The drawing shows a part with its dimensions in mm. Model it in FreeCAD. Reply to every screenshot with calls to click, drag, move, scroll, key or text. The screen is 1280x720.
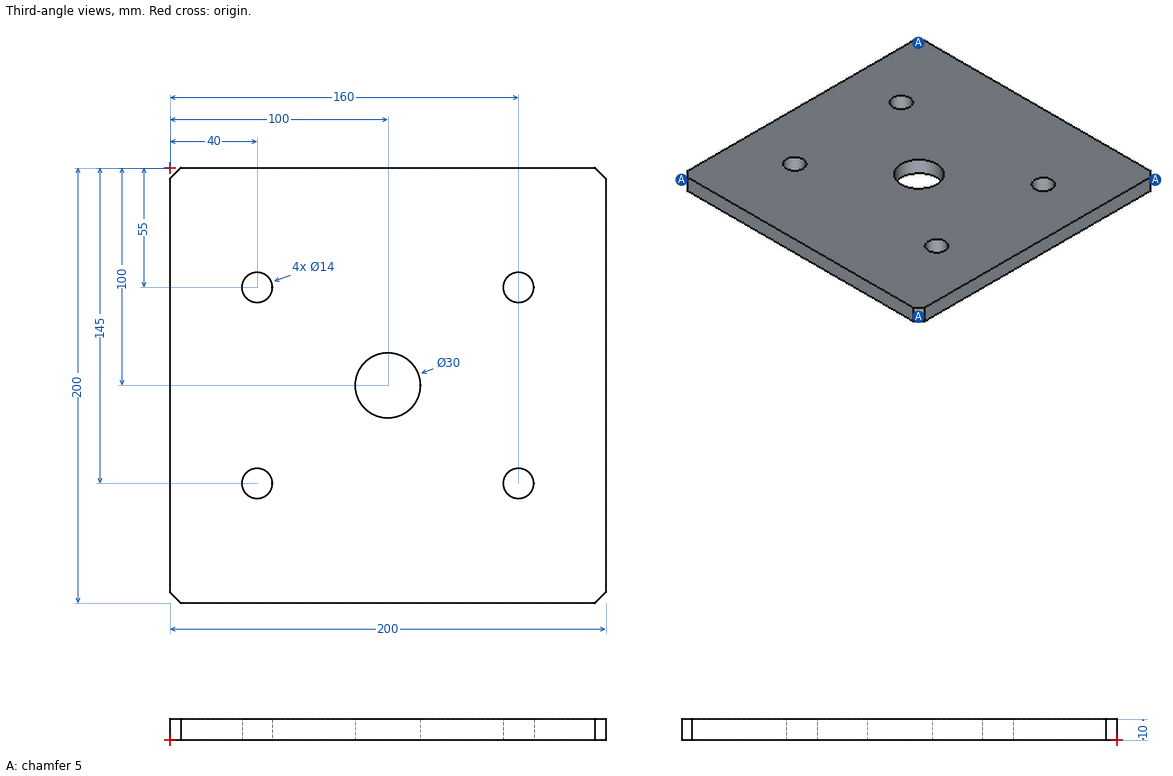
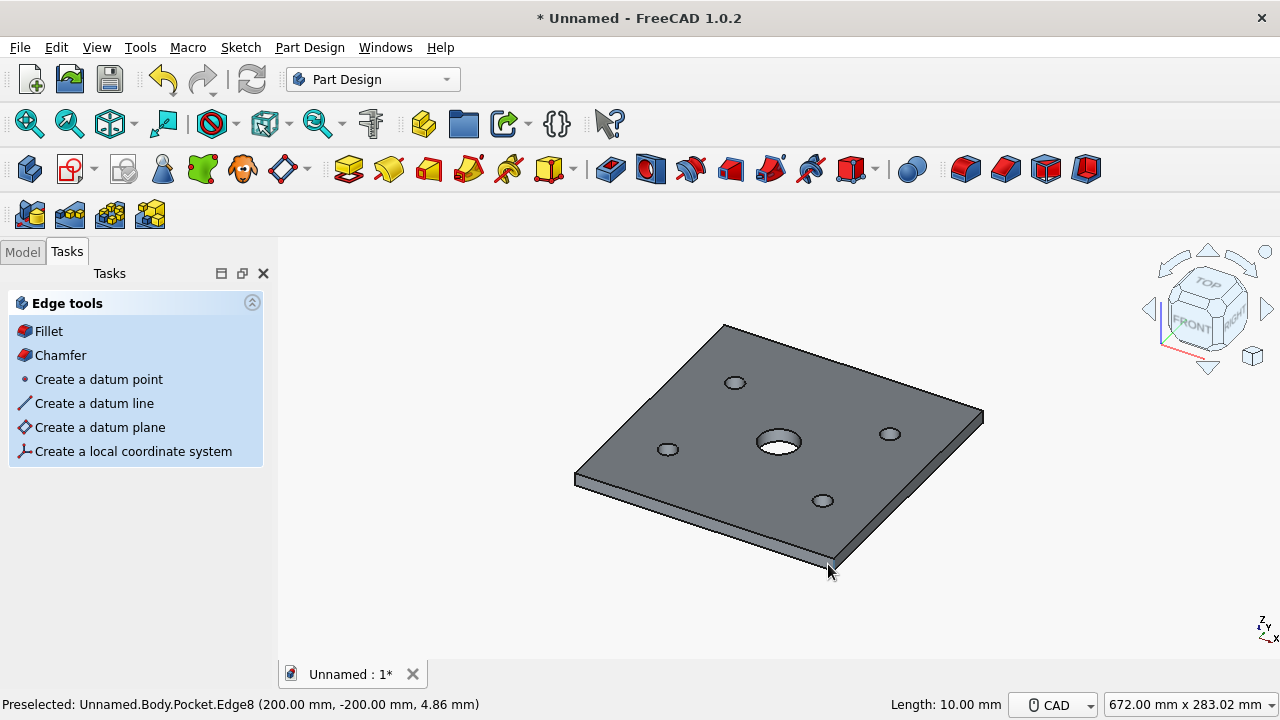
scroll(724, 330, up, 5)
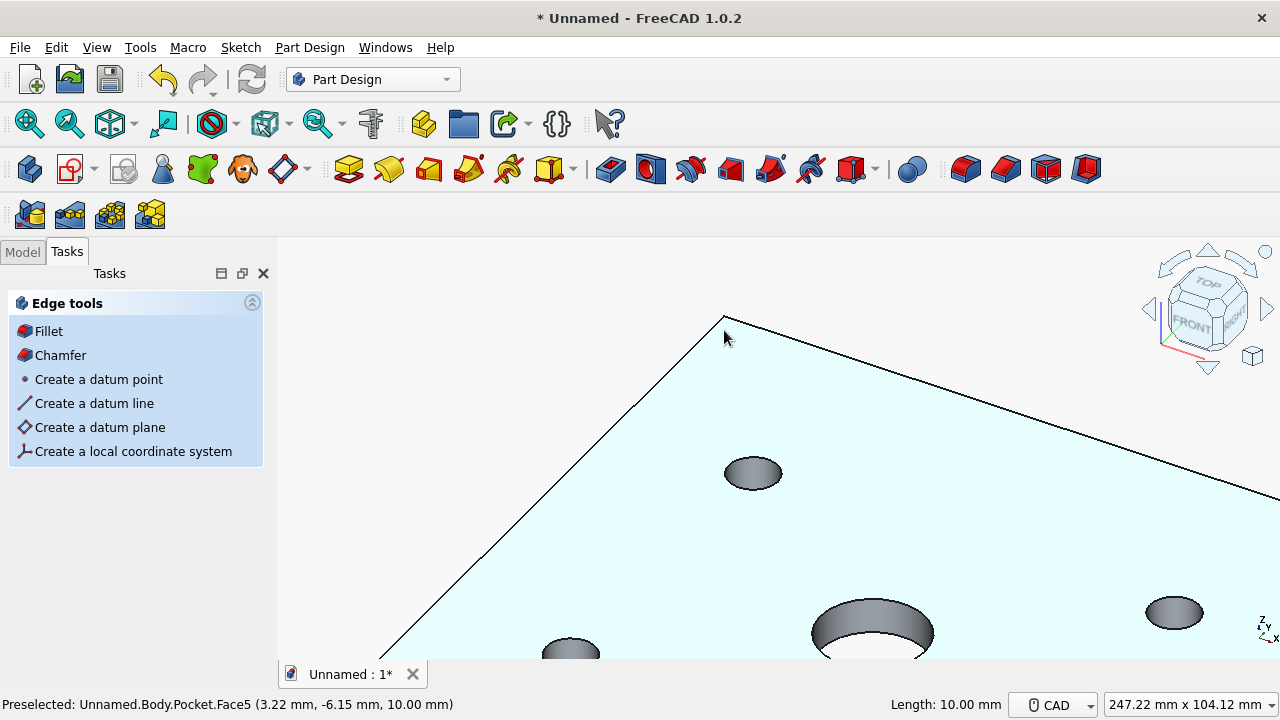
click(30, 124)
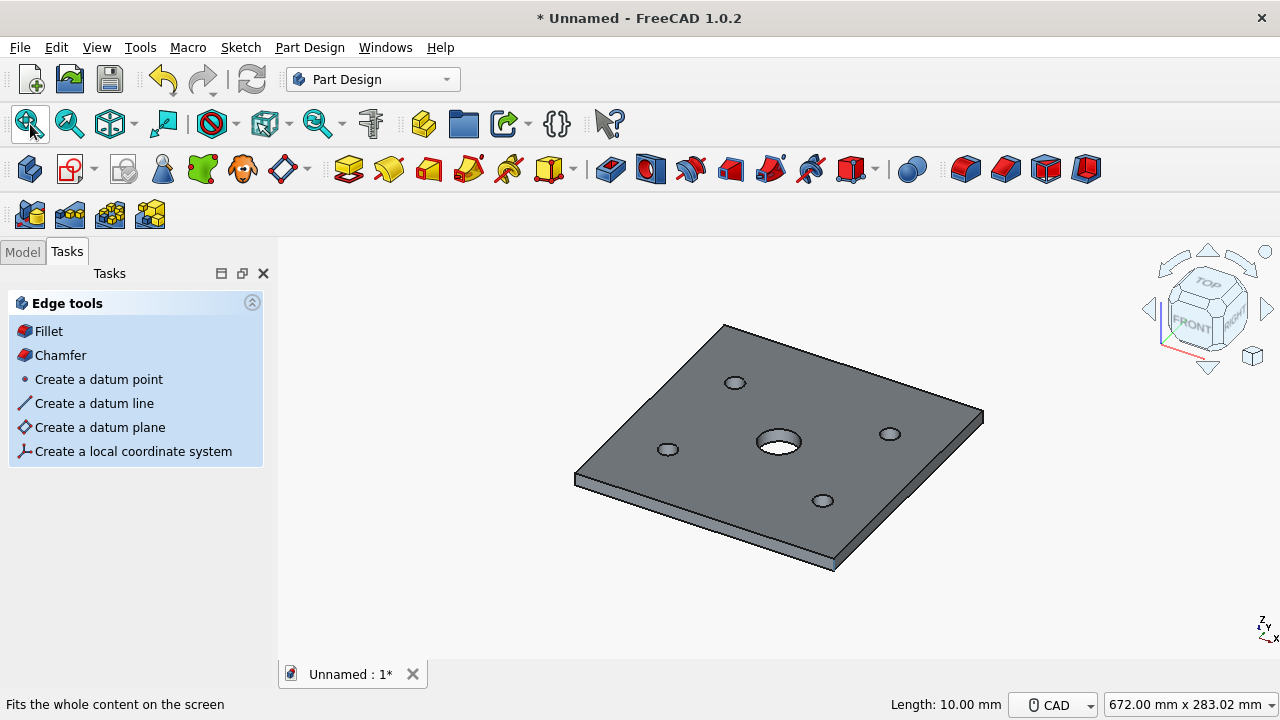
key(0)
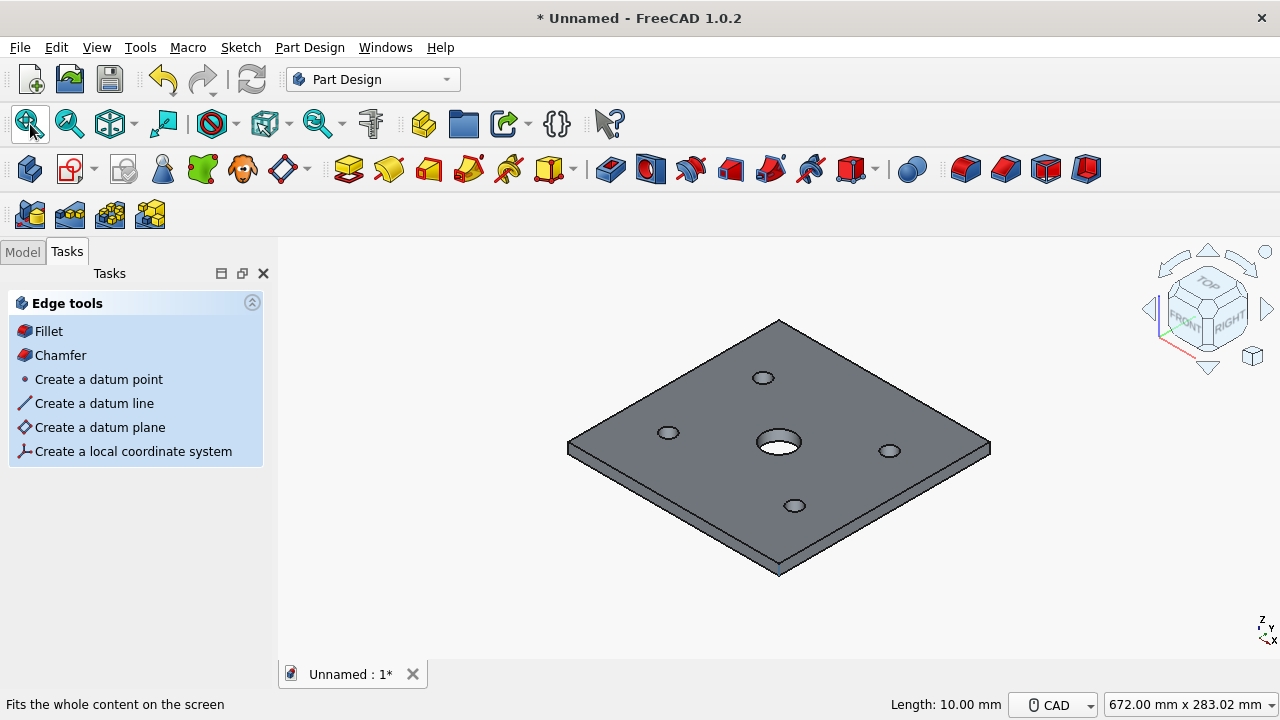
scroll(779, 325, up, 5)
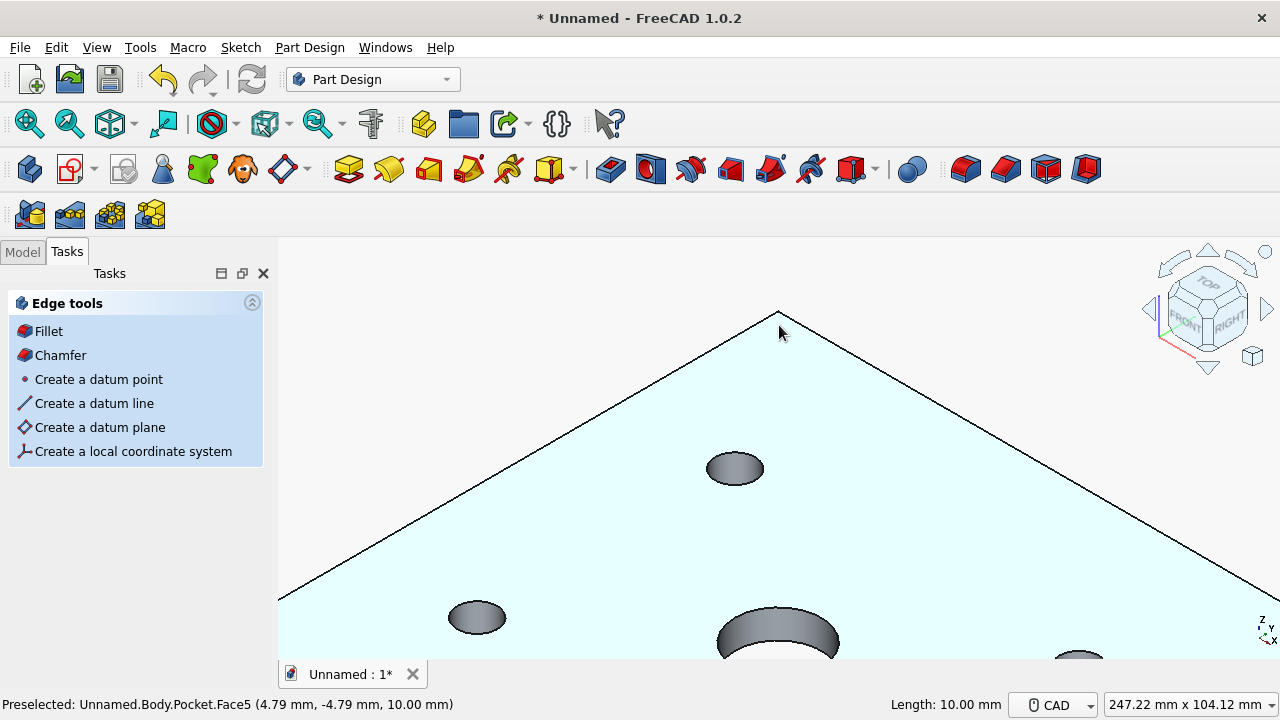
click(30, 124)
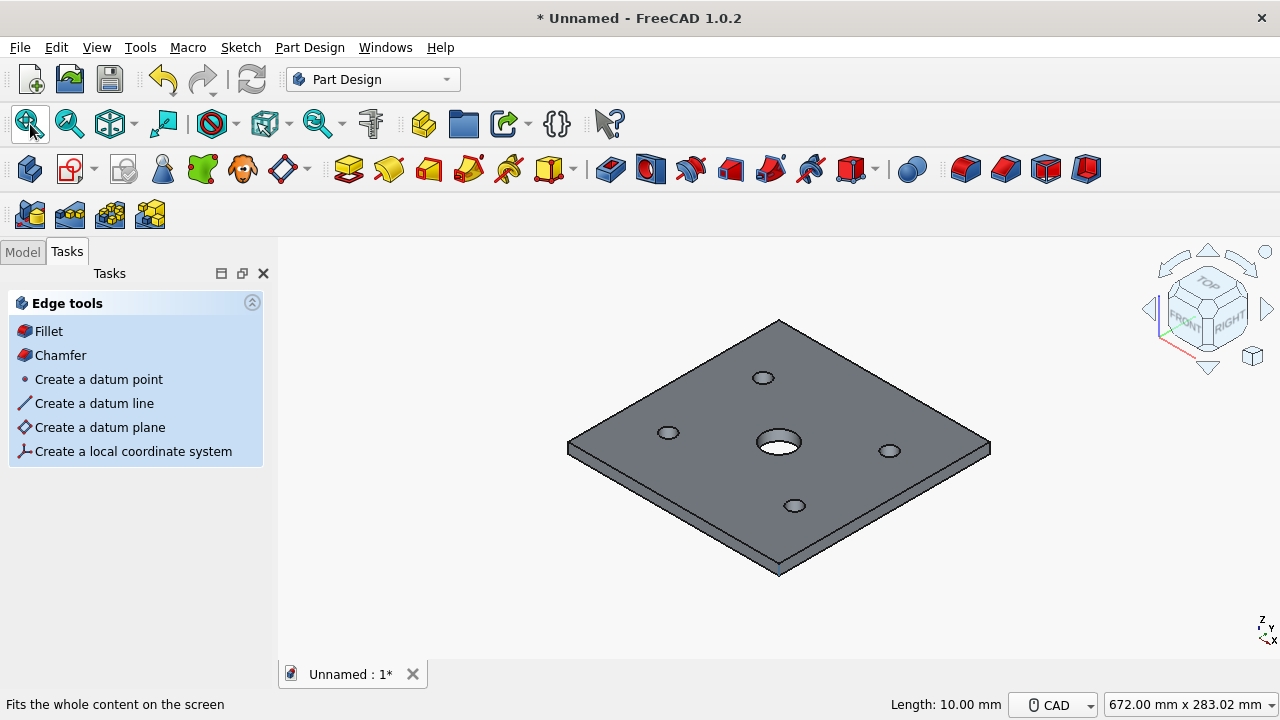
key(2)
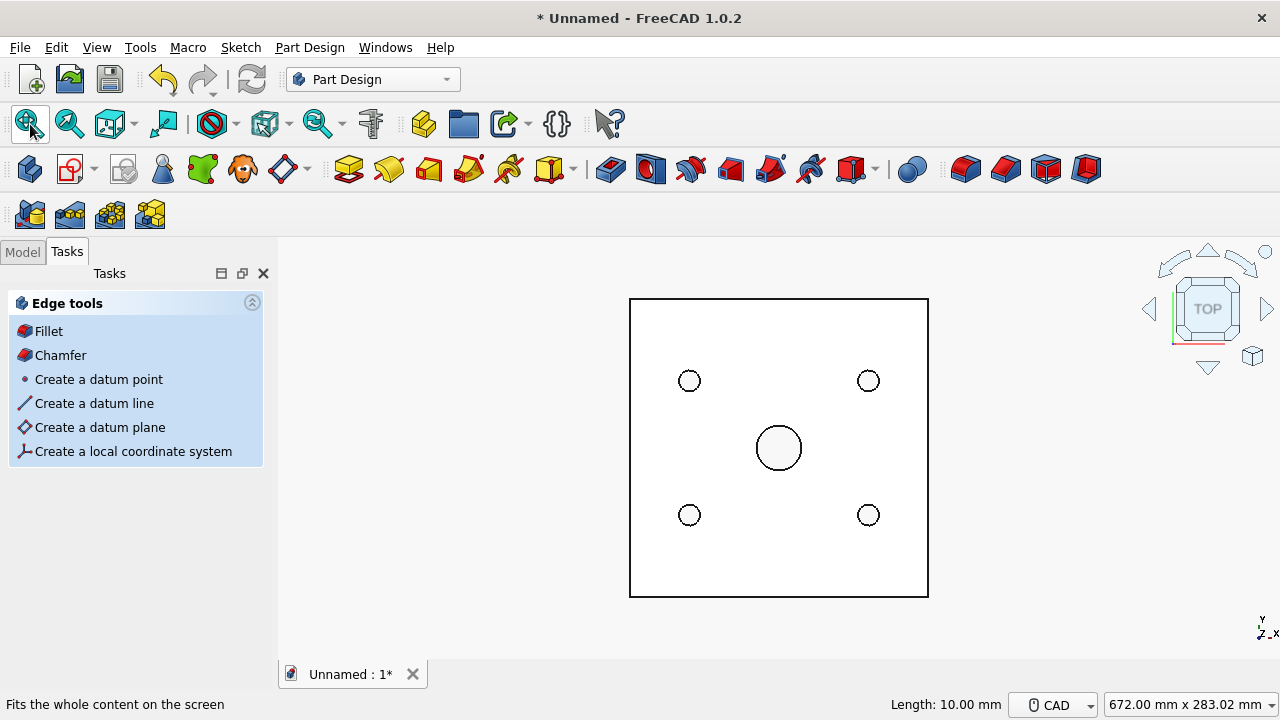
scroll(630, 298, up, 5)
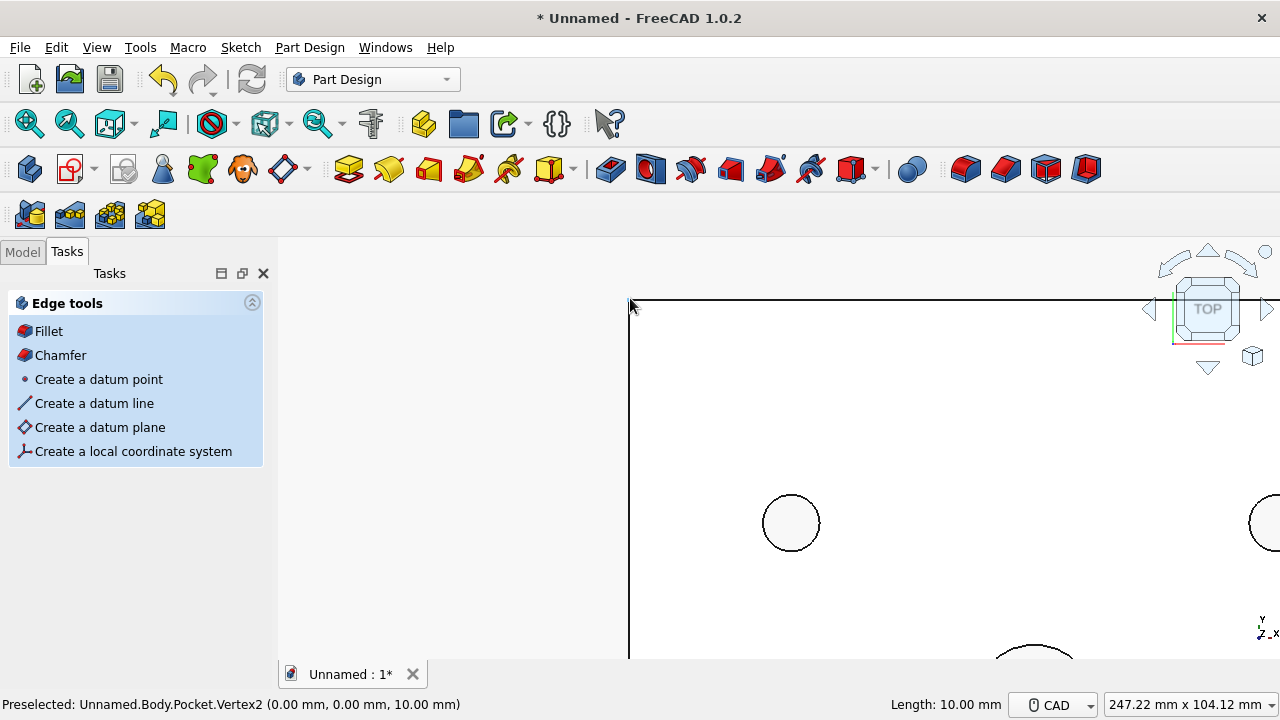
click(30, 124)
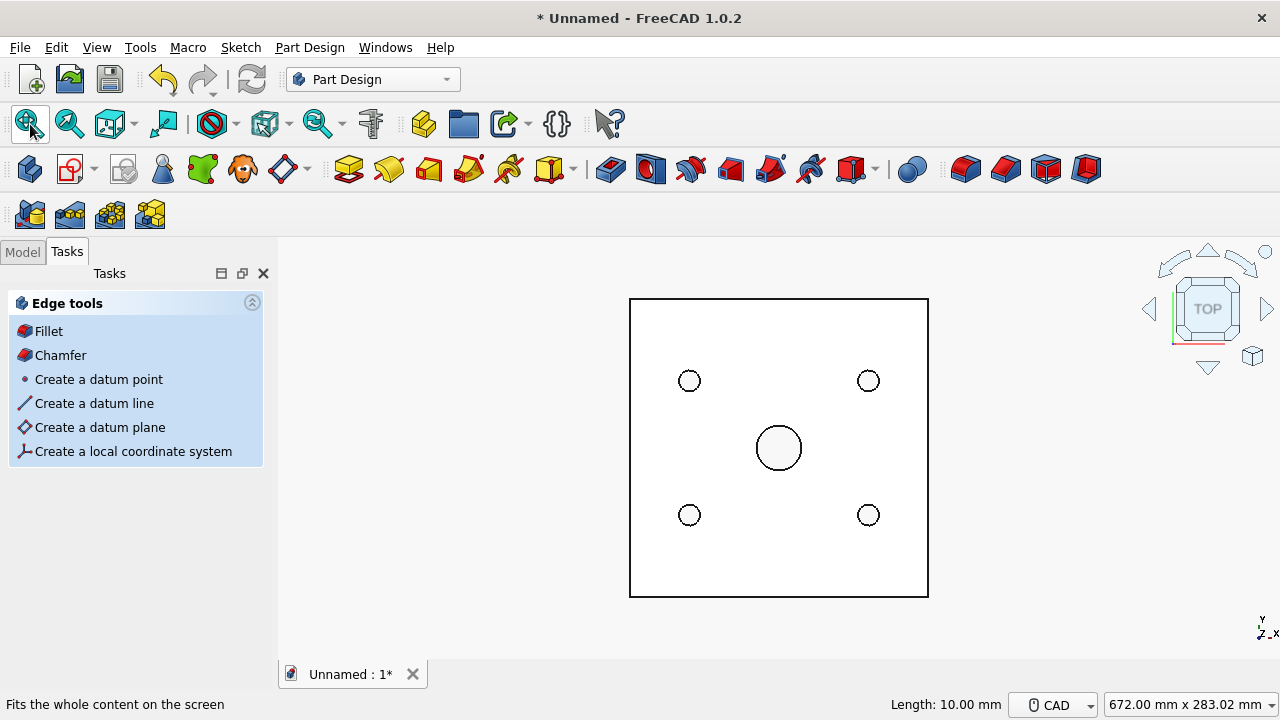
key(1)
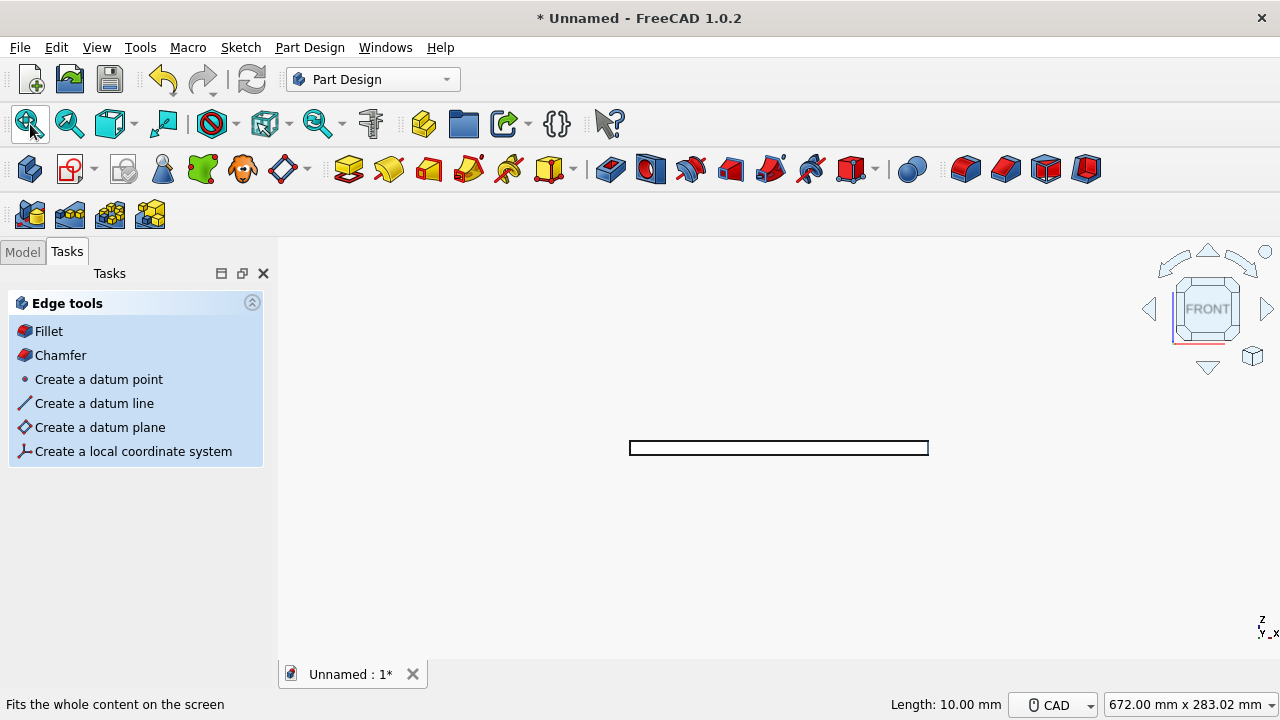
click(30, 124)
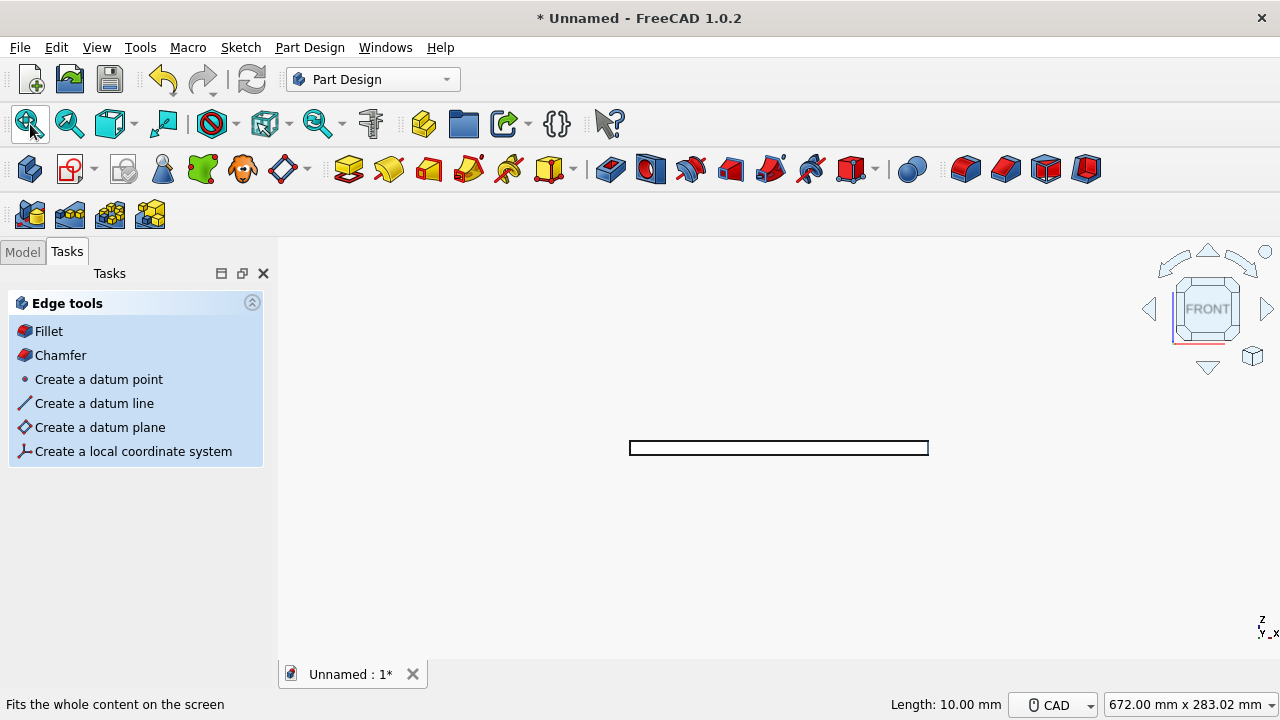
click(630, 447, ctrl)